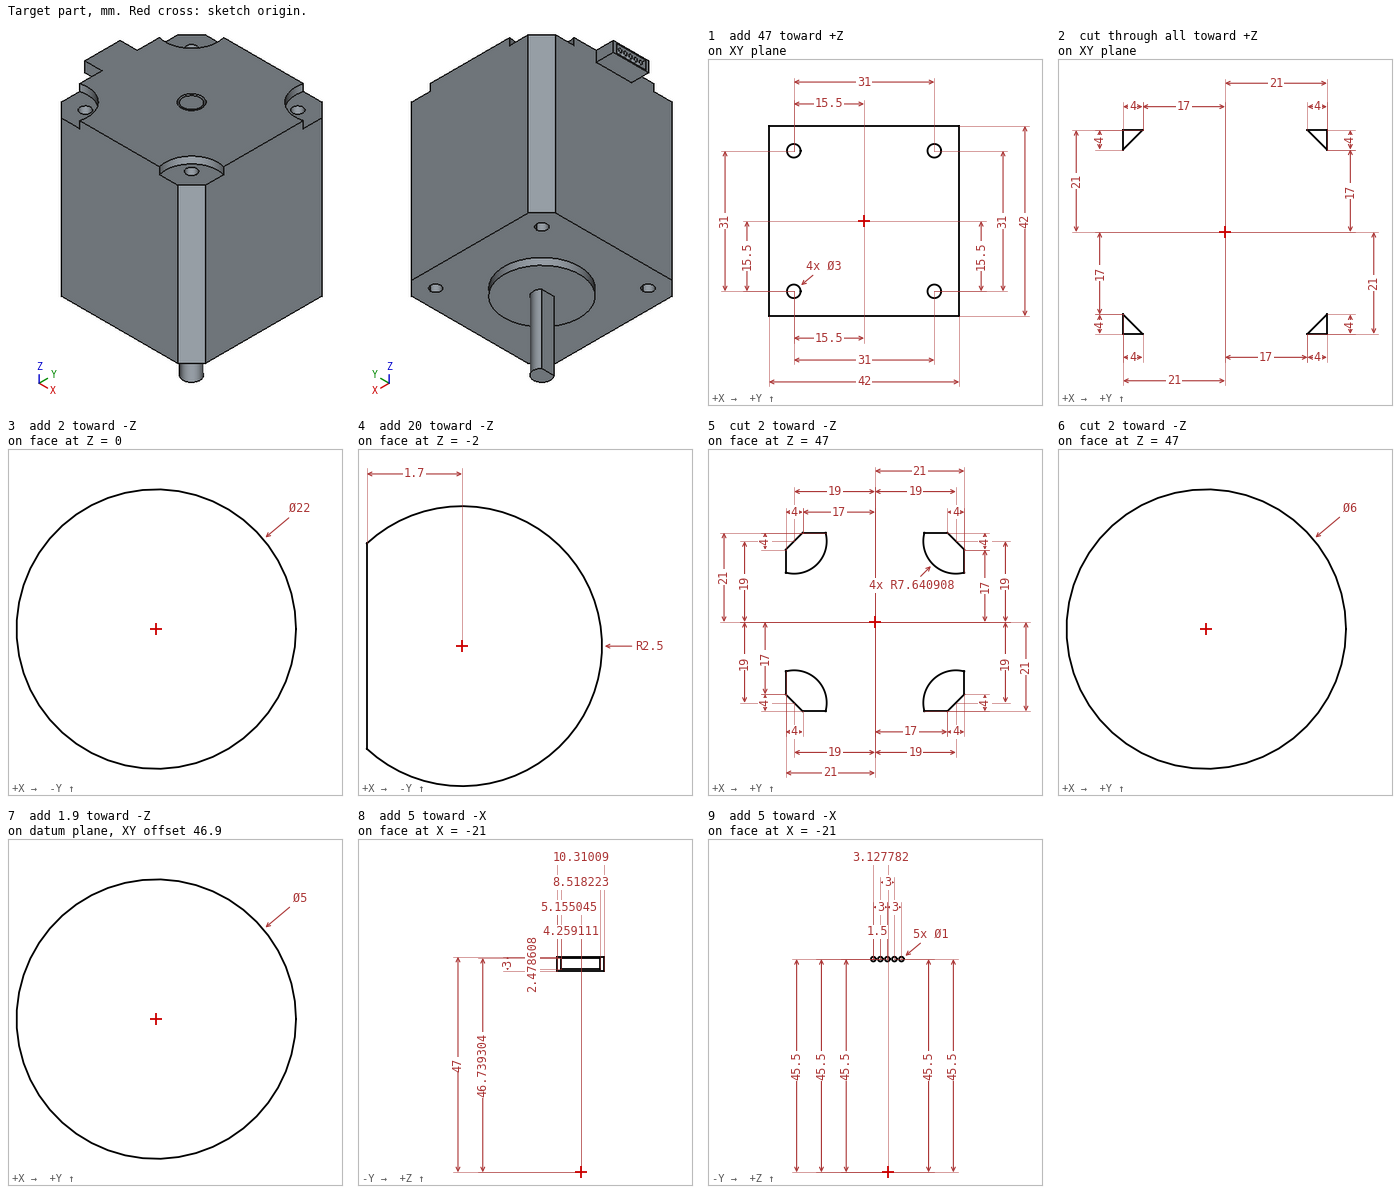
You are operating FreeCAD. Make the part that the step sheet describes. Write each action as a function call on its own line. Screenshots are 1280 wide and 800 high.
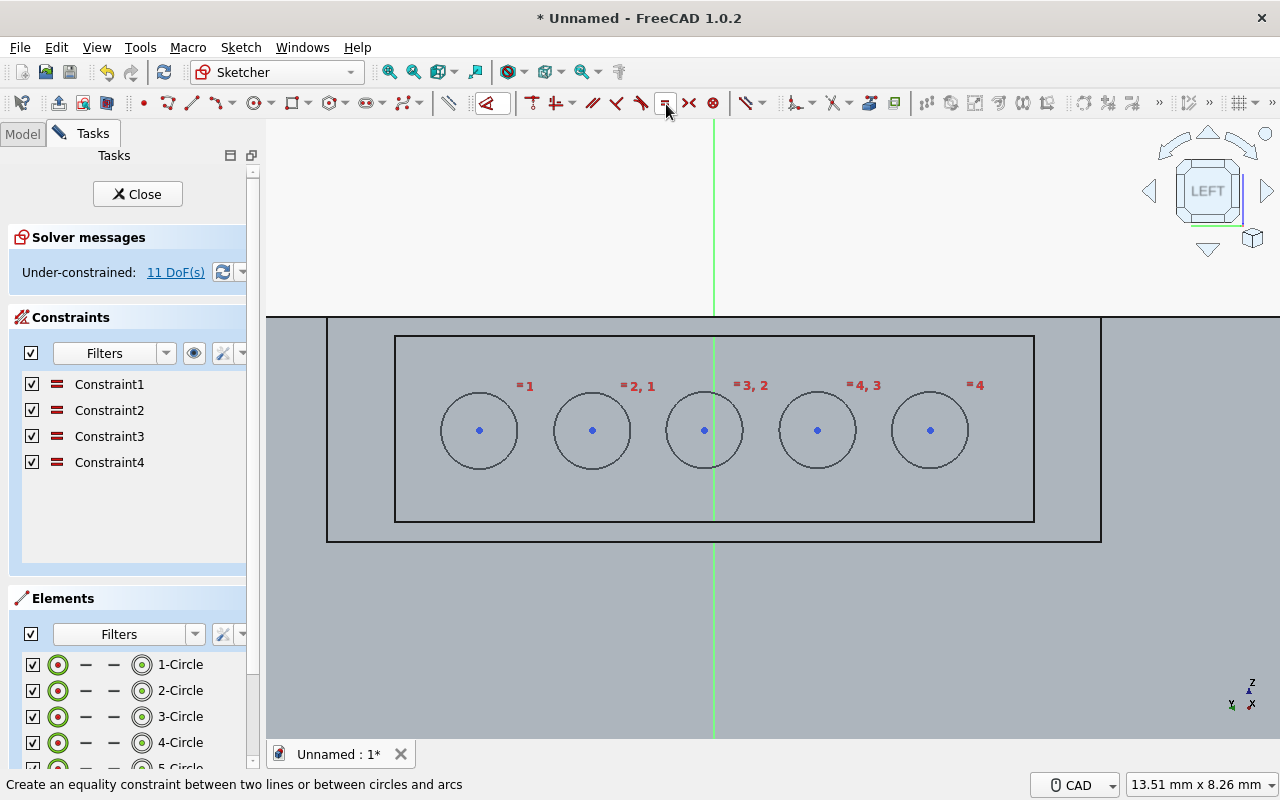
click(506, 404)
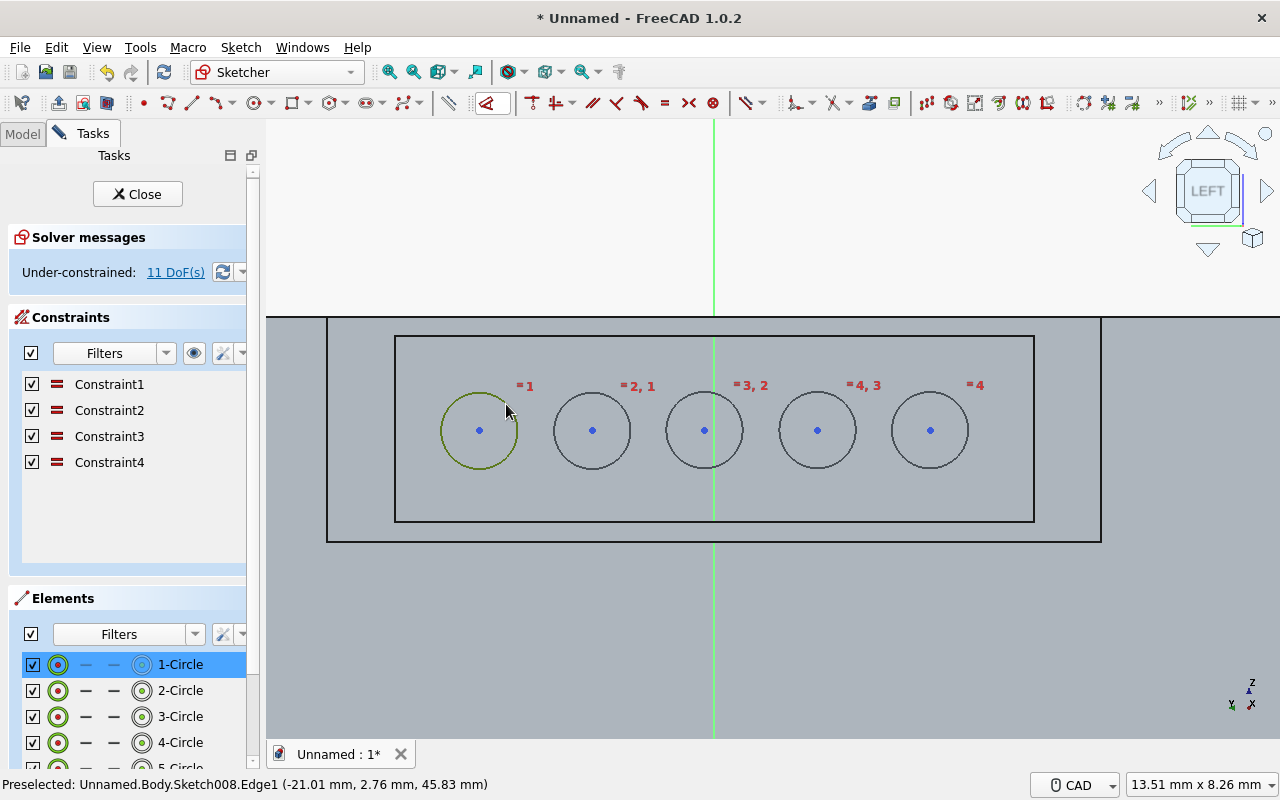
key(k)
key(o)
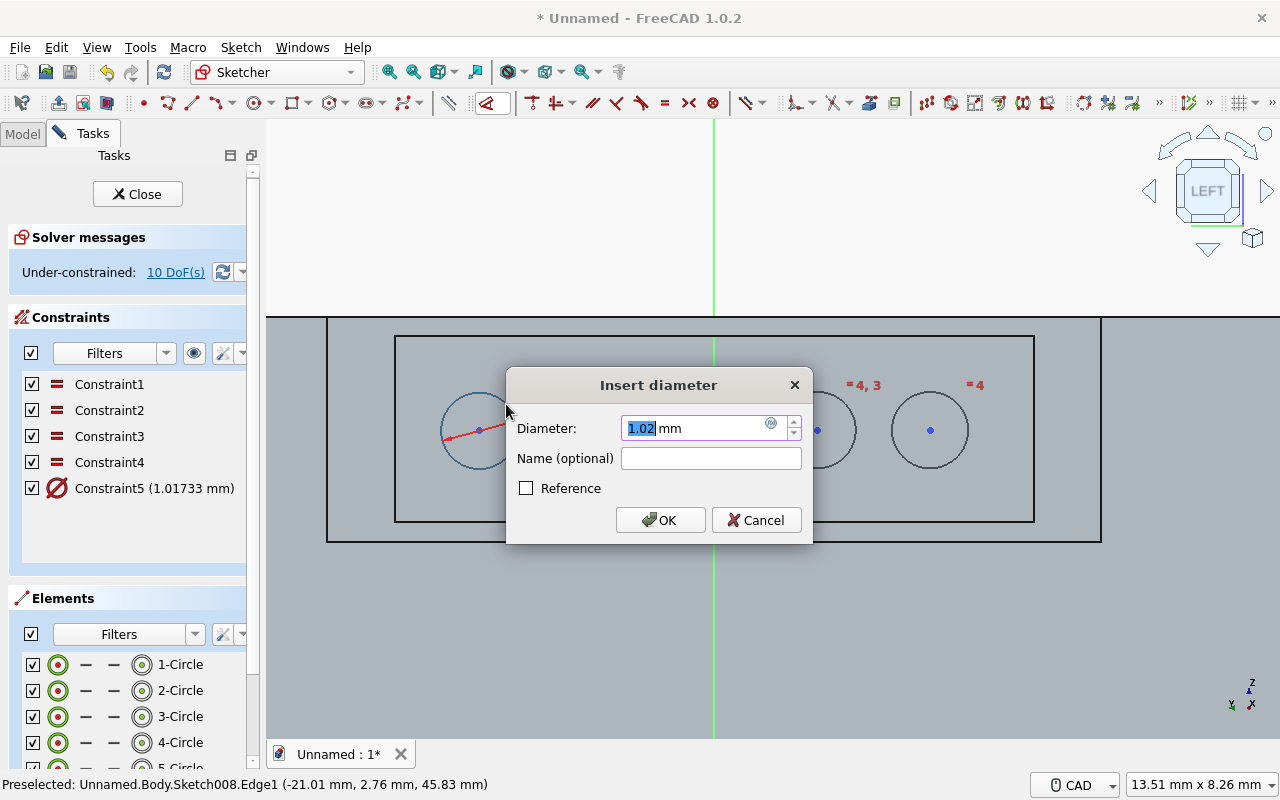
text(1)
key(Return)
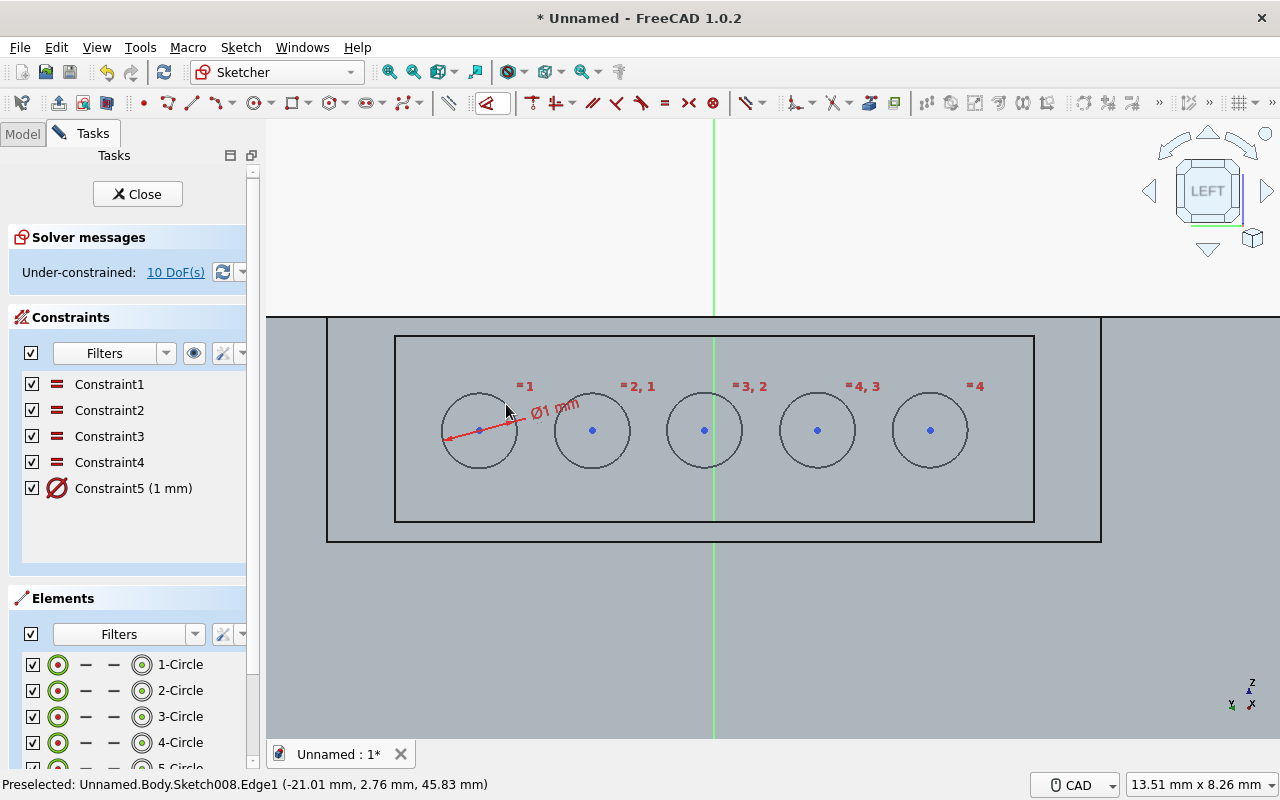
click(479, 431)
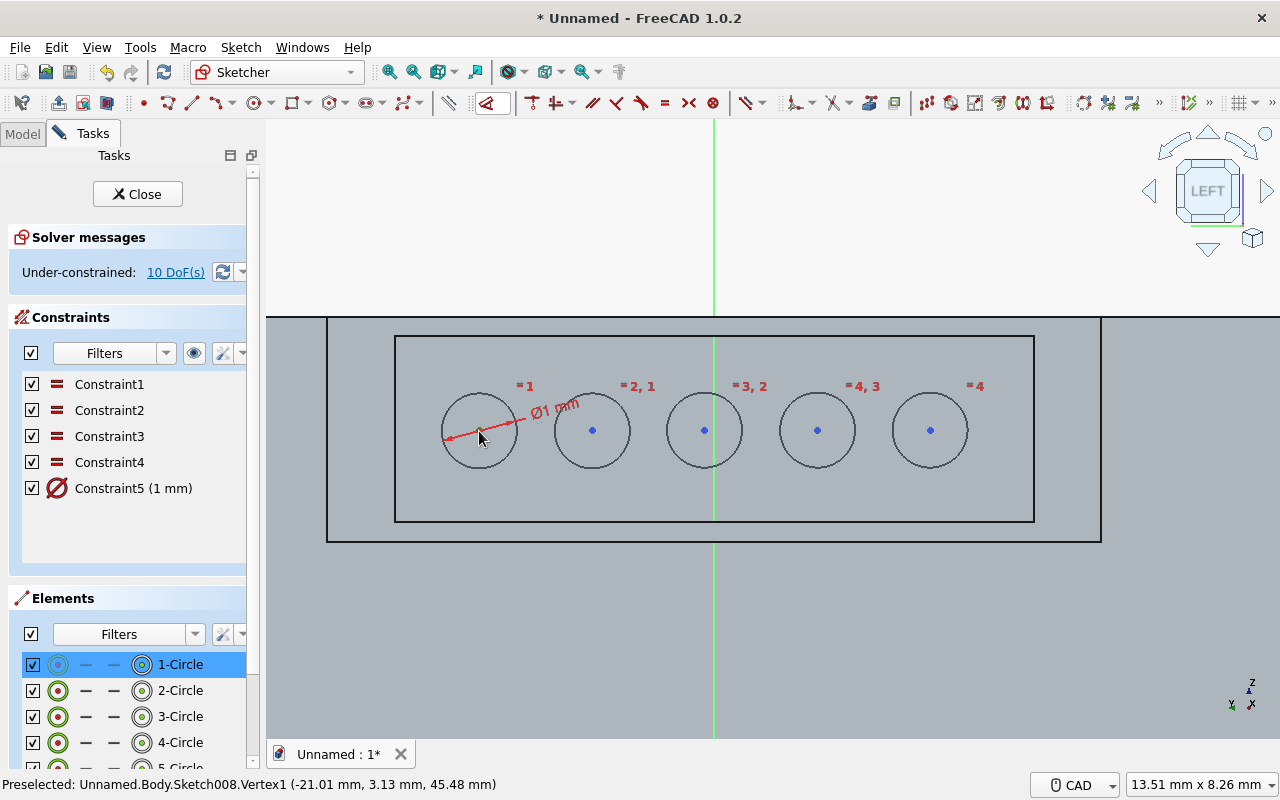
click(705, 430)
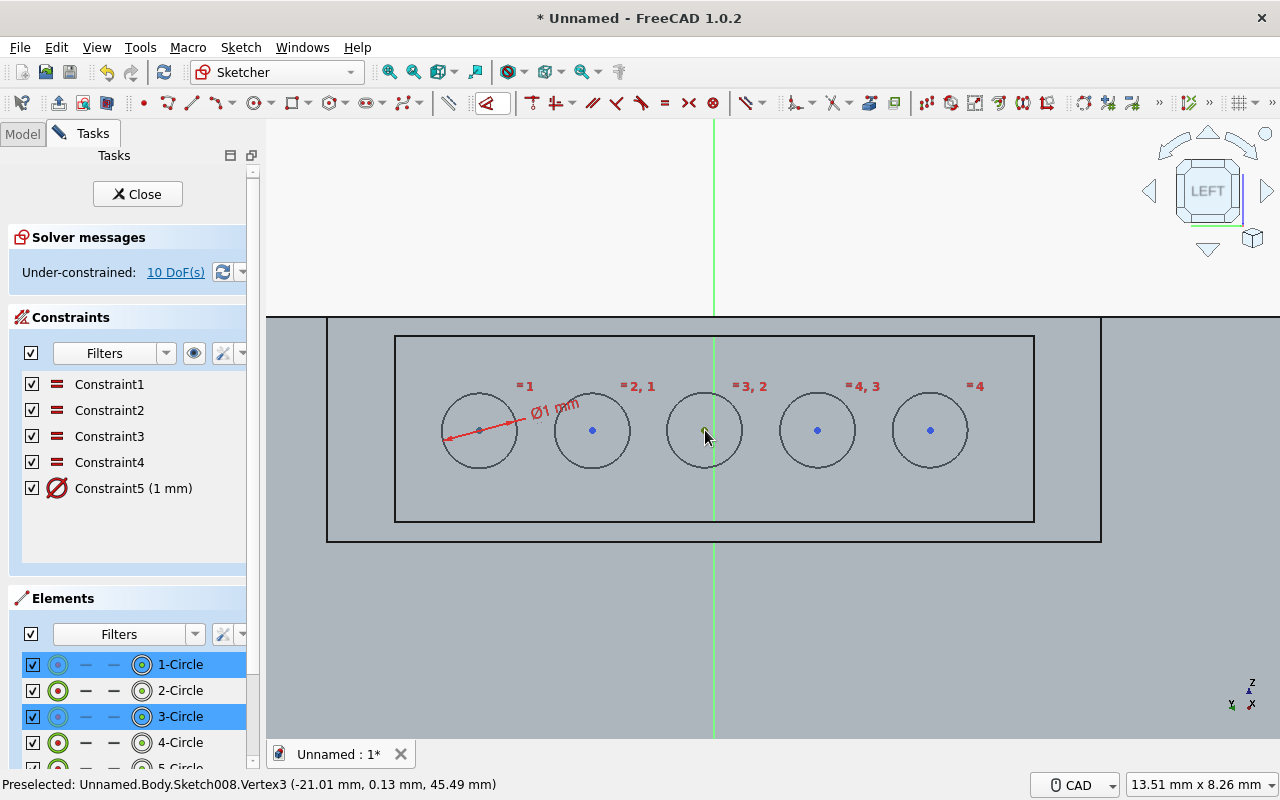
click(504, 104)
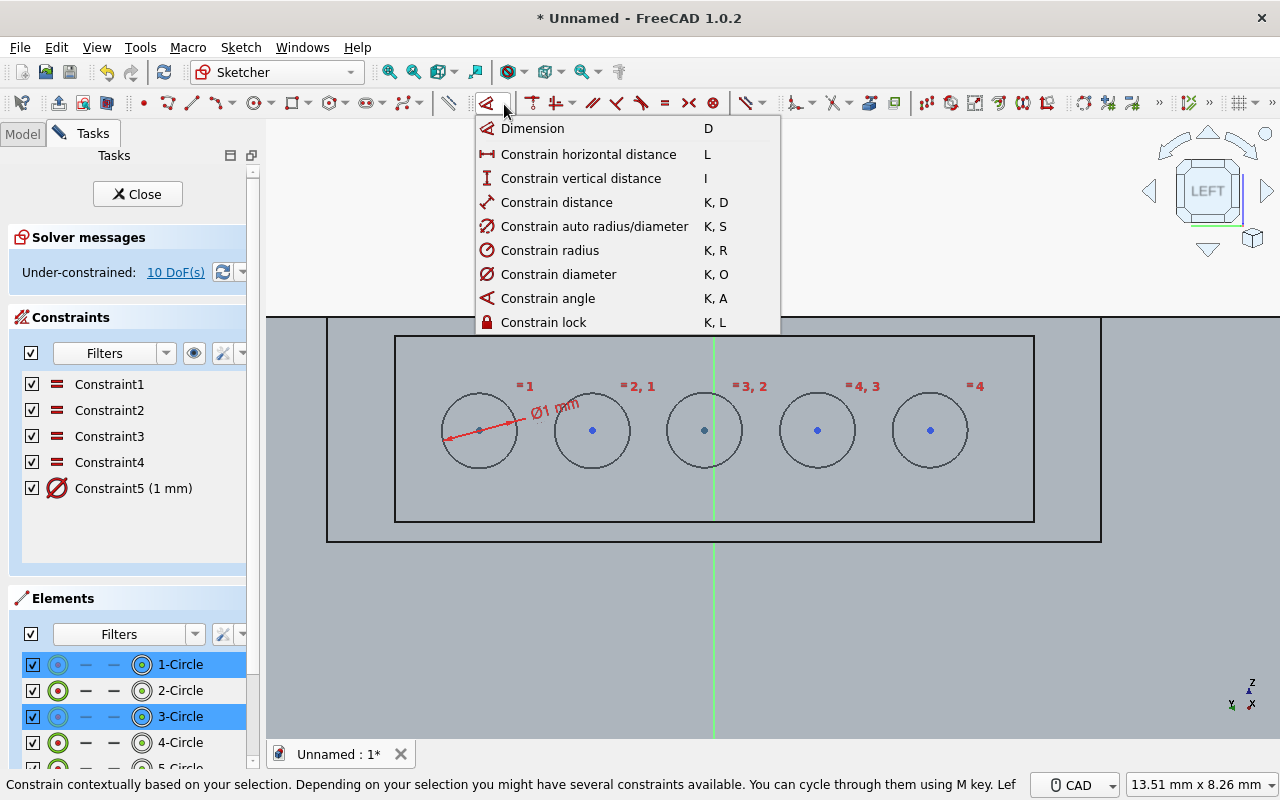
click(628, 154)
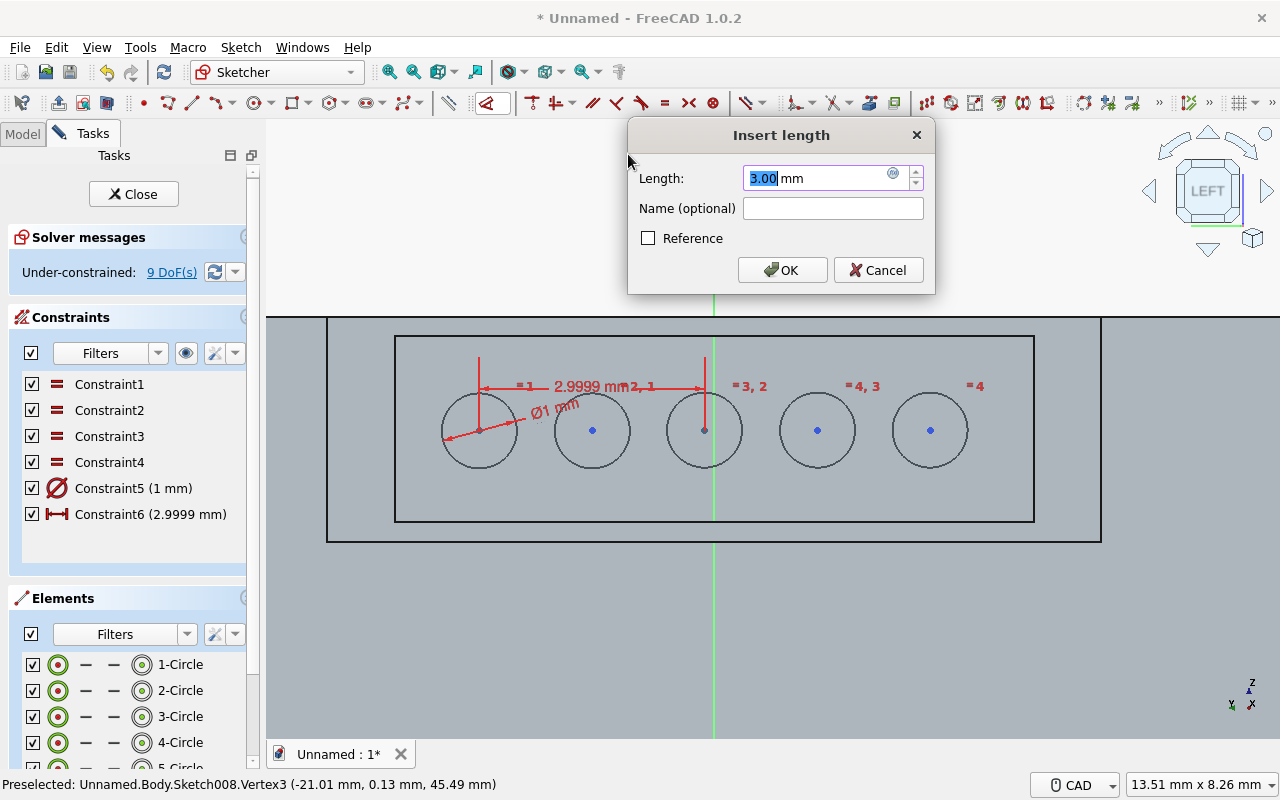
text(3)
key(Return)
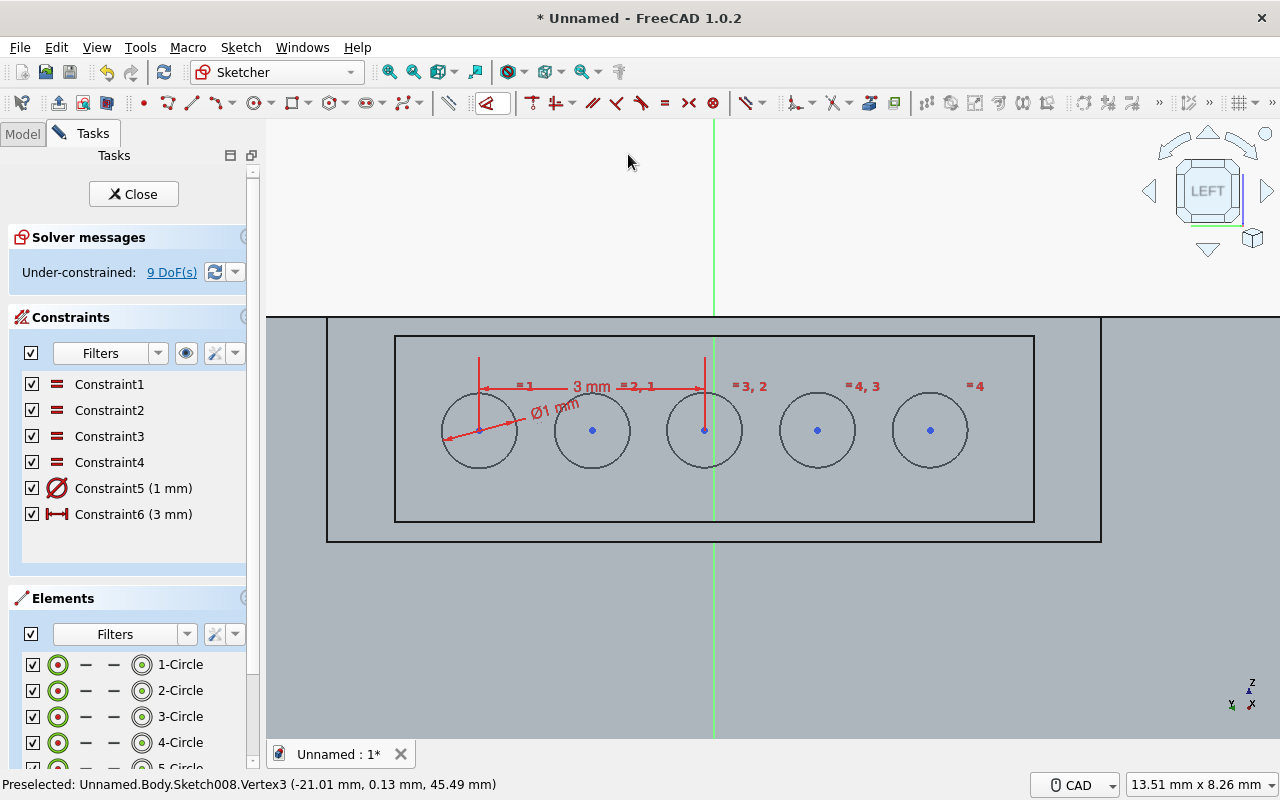
click(592, 431)